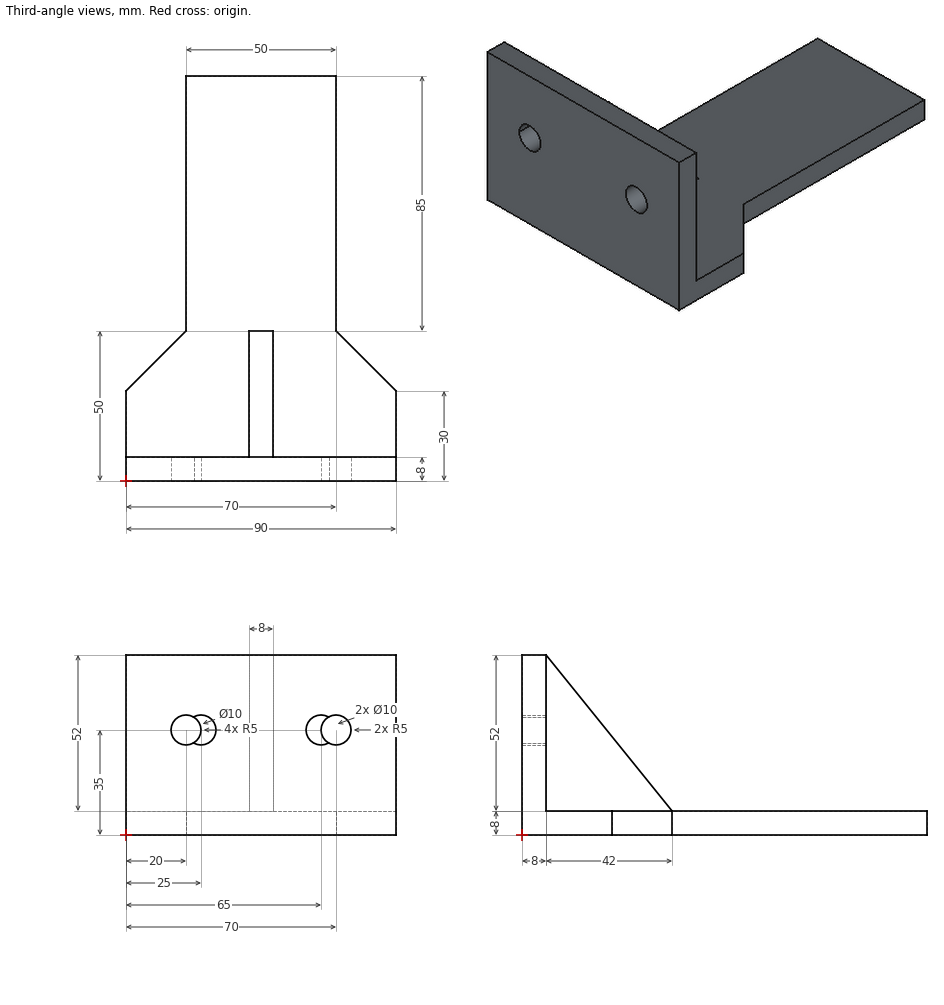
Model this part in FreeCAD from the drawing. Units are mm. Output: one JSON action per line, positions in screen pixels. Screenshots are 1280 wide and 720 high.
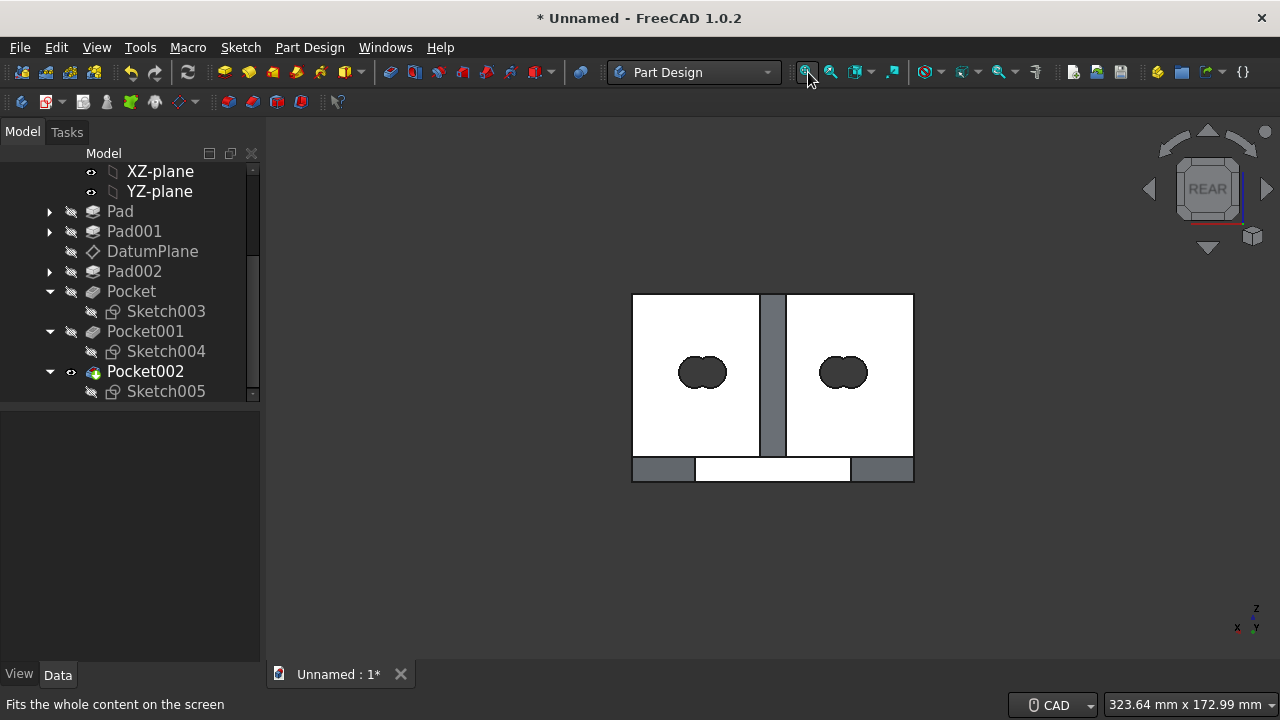
{"action": "left_click", "coordinate": [678, 421]}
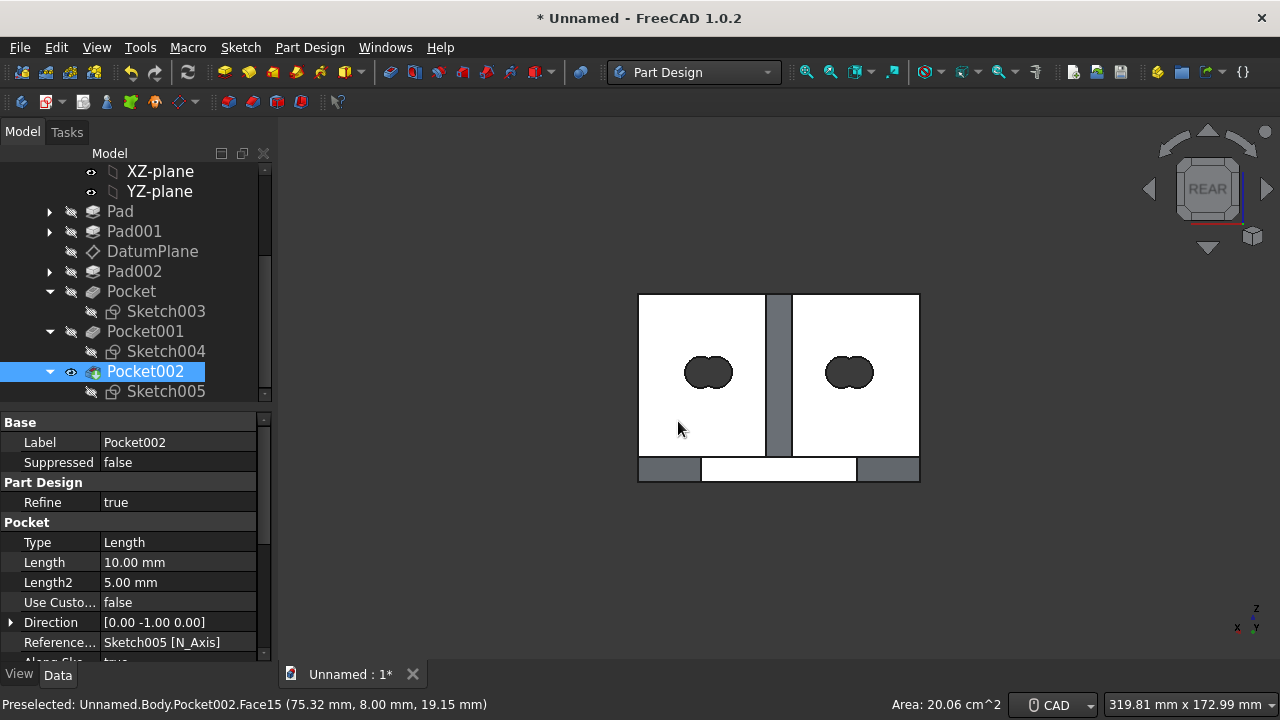
{"action": "left_click", "coordinate": [46, 102]}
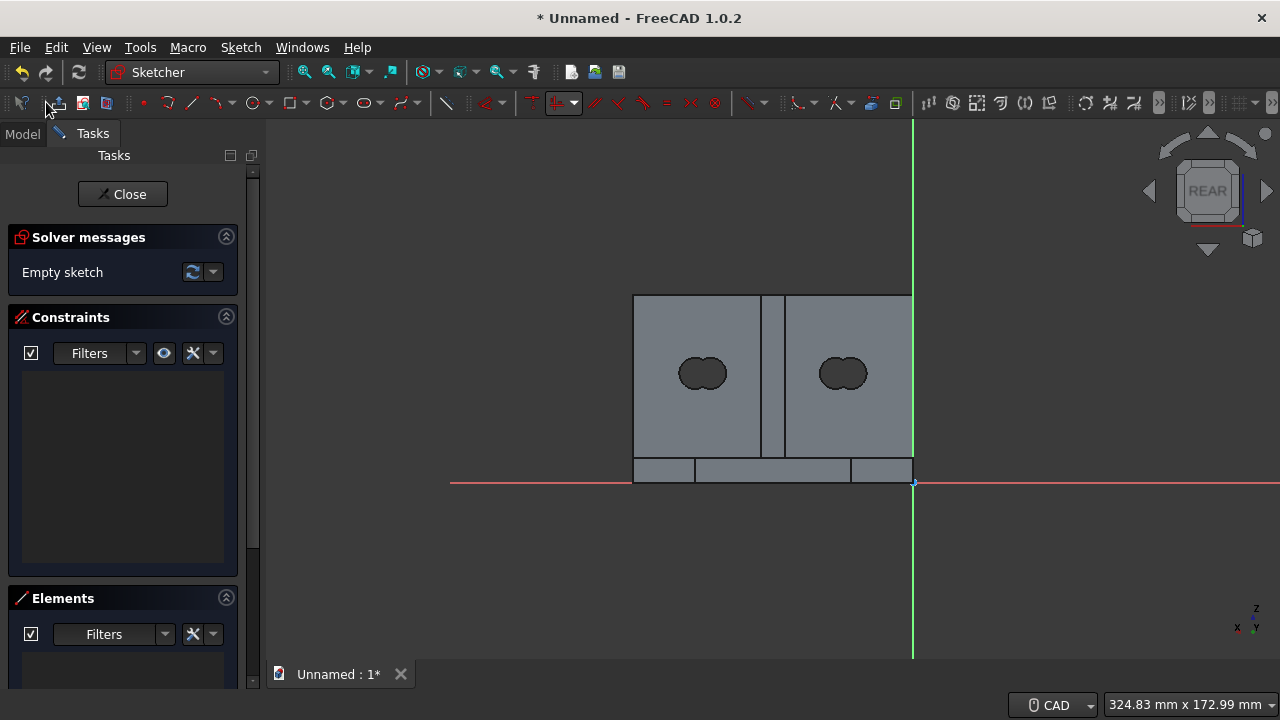
{"action": "left_click", "coordinate": [108, 104]}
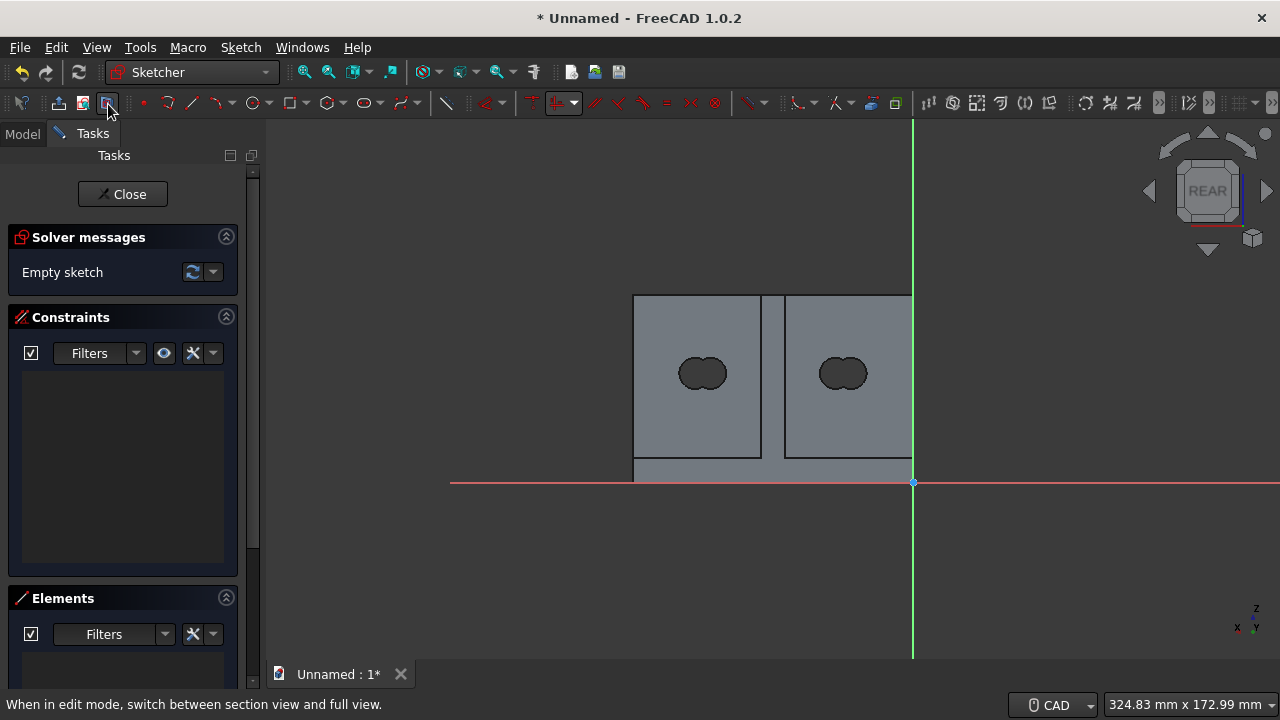
{"action": "scroll", "coordinate": [868, 440], "scroll_direction": "up", "scroll_amount": 5}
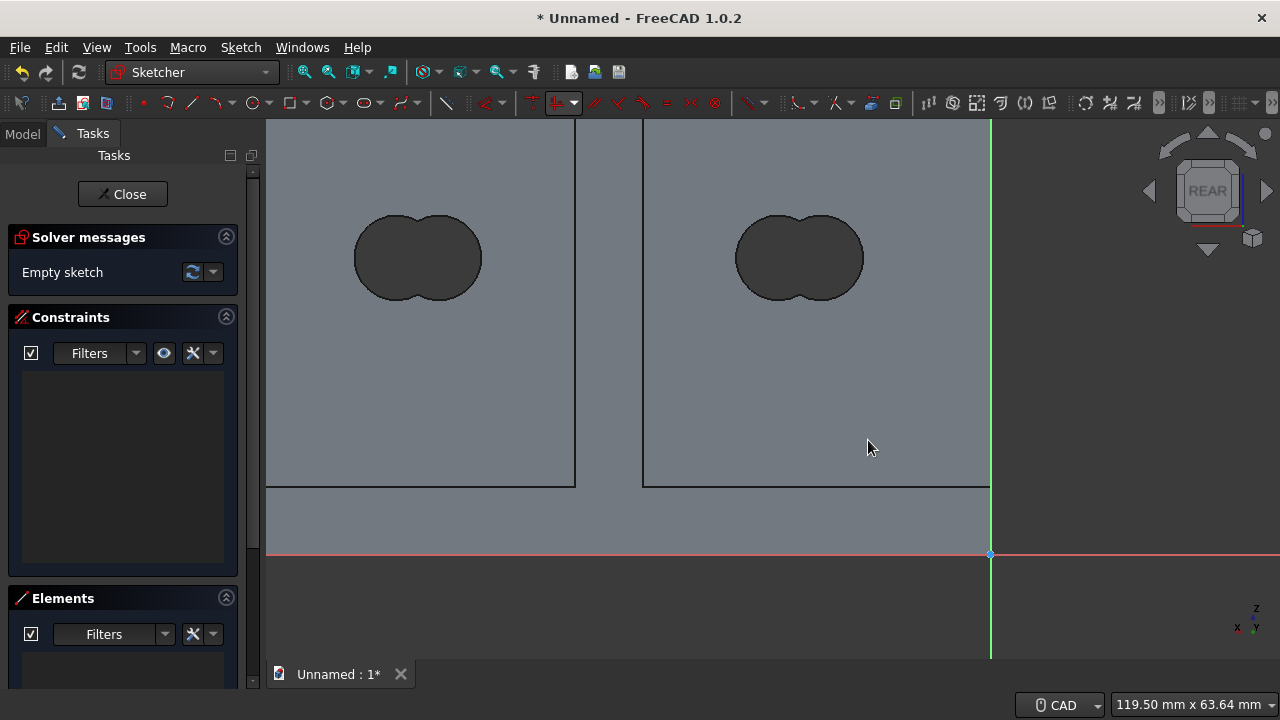
{"action": "left_click", "coordinate": [216, 104]}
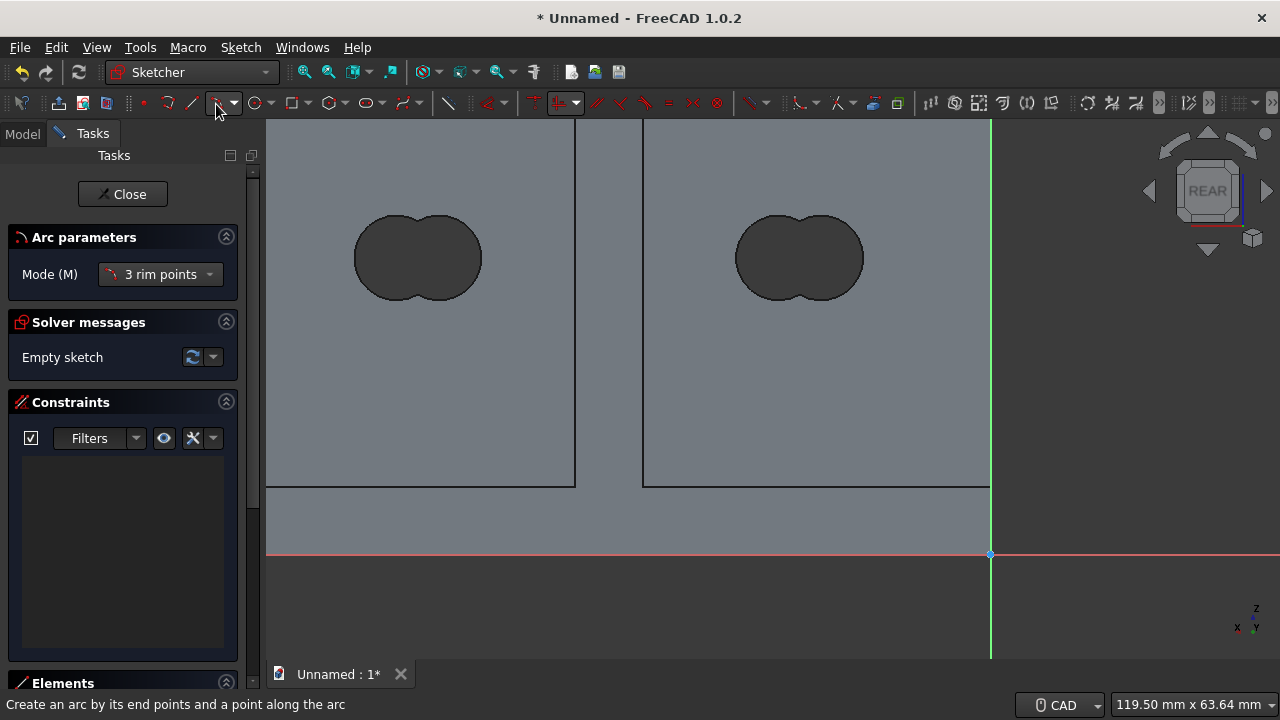
{"action": "left_click", "coordinate": [800, 295]}
{"action": "left_click", "coordinate": [800, 221]}
{"action": "left_click", "coordinate": [736, 258]}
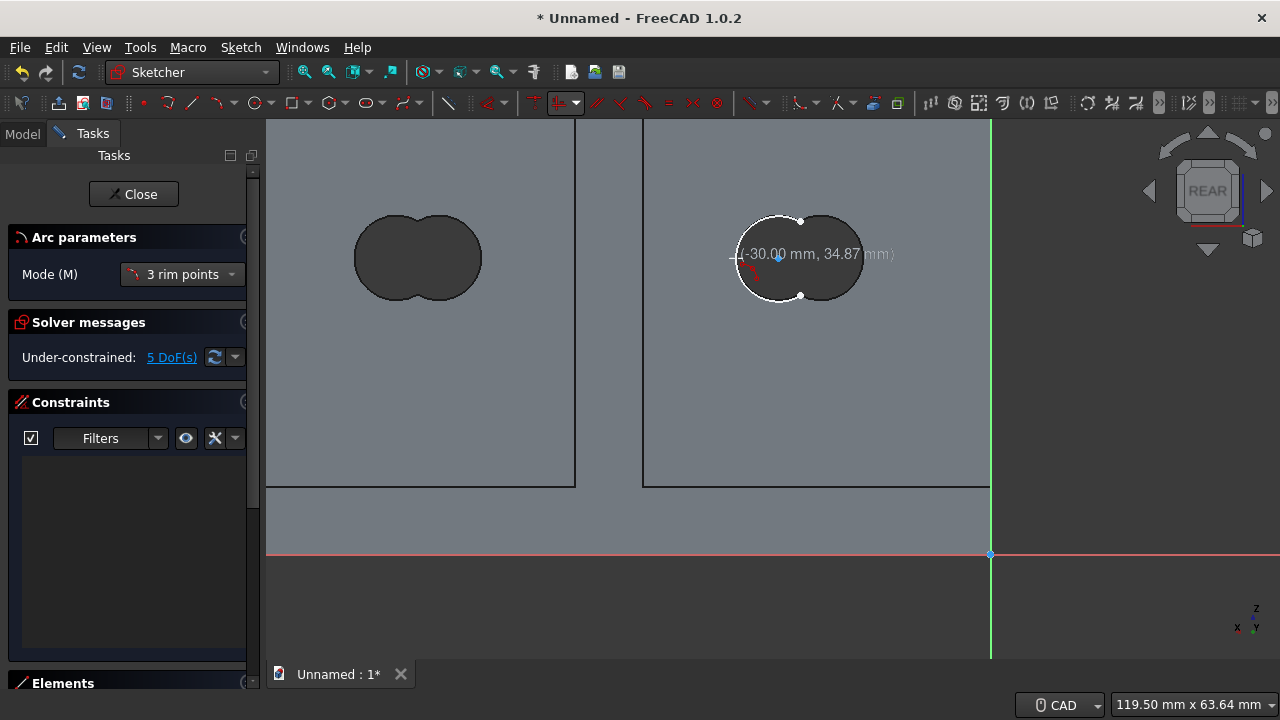
{"action": "left_click", "coordinate": [800, 222]}
{"action": "left_click", "coordinate": [800, 296]}
{"action": "left_click", "coordinate": [778, 258]}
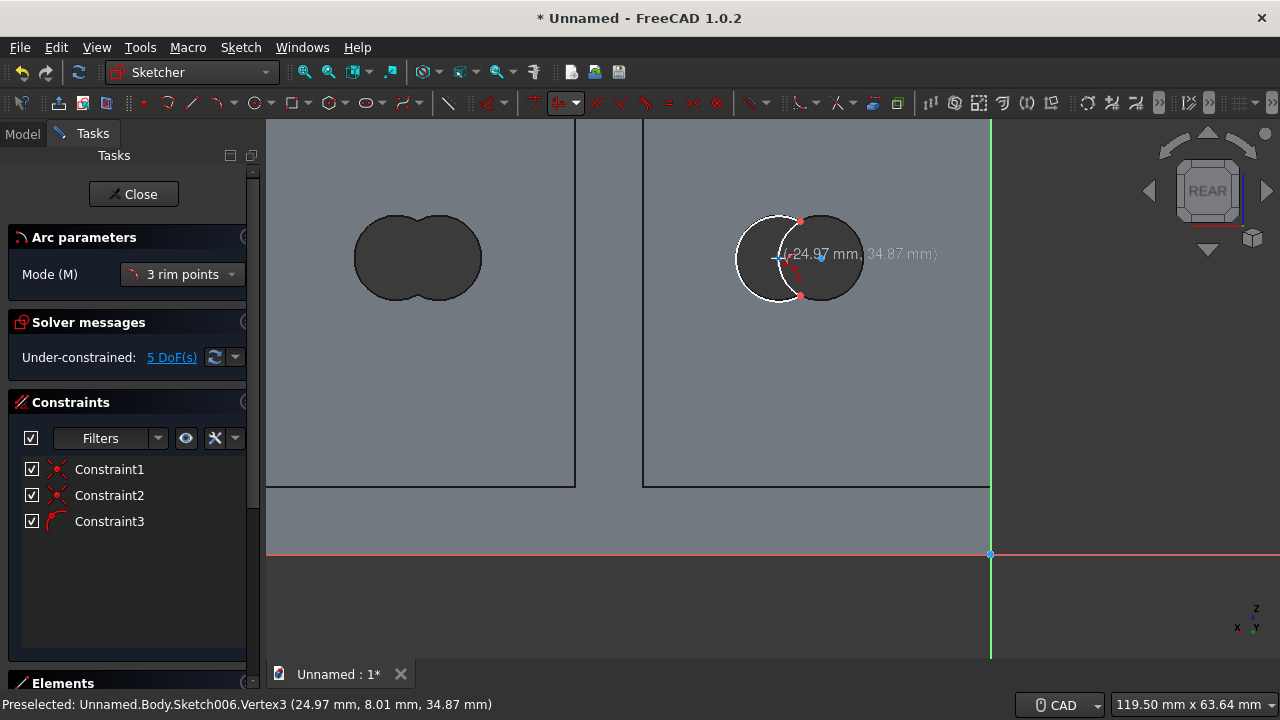
{"action": "left_click", "coordinate": [418, 295]}
{"action": "left_click", "coordinate": [418, 221]}
{"action": "left_click", "coordinate": [439, 258]}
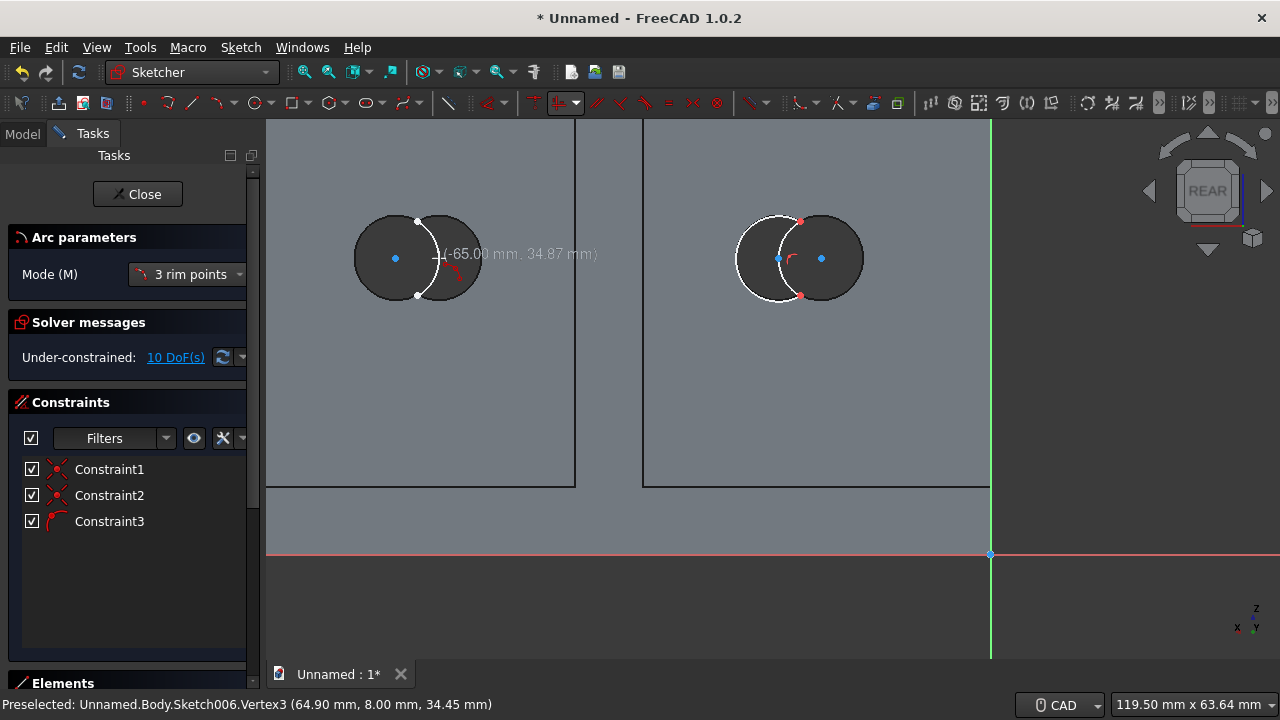
{"action": "left_click", "coordinate": [418, 222]}
{"action": "left_click", "coordinate": [418, 296]}
{"action": "left_click", "coordinate": [481, 258]}
{"action": "key", "text": "Escape"}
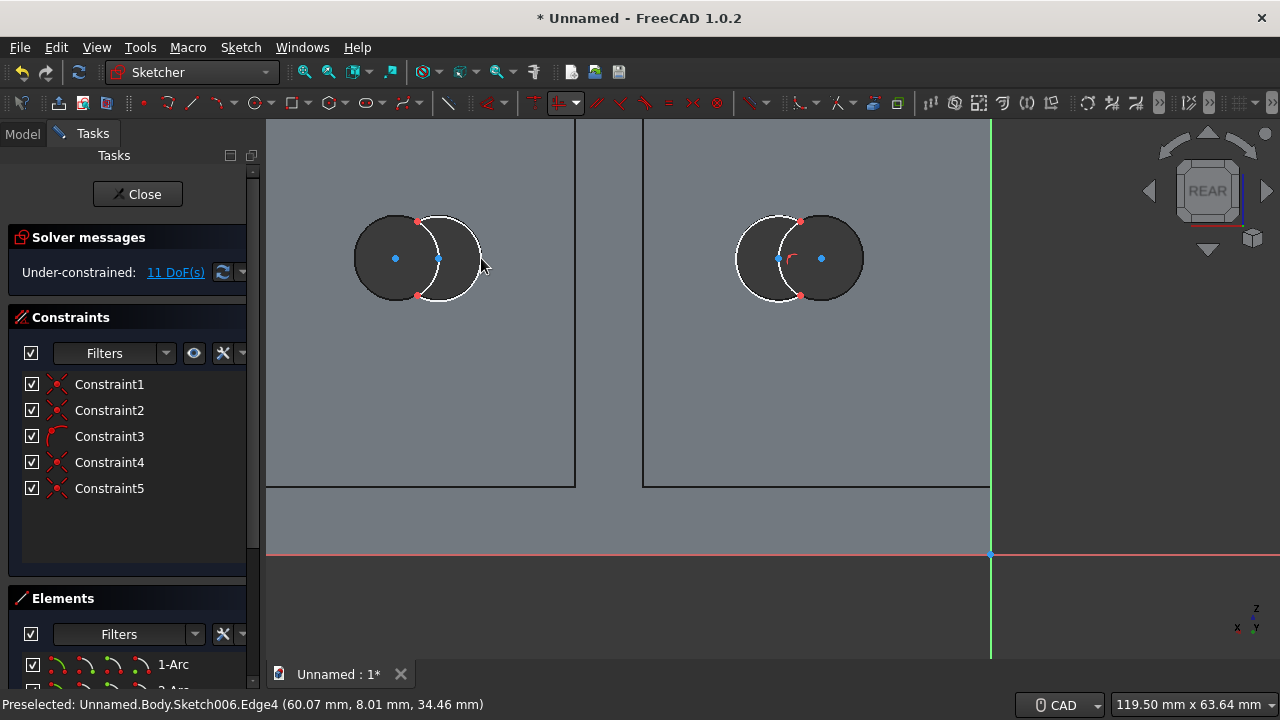
{"action": "left_click", "coordinate": [750, 227]}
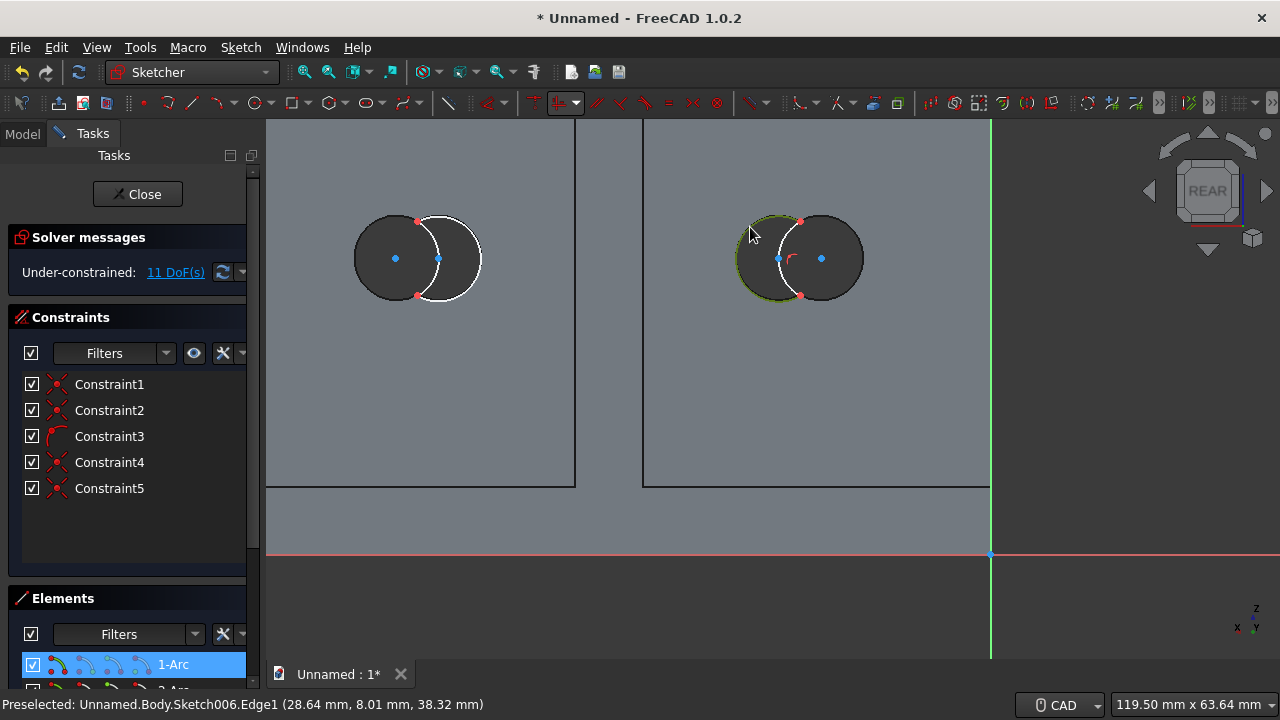
{"action": "left_click", "coordinate": [782, 242]}